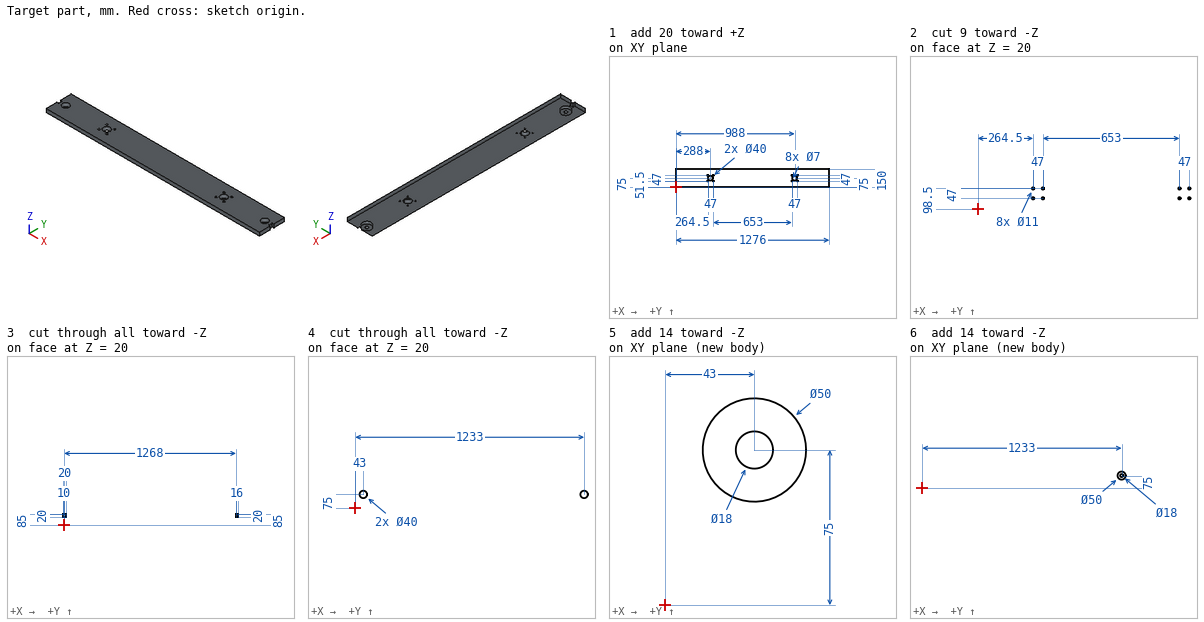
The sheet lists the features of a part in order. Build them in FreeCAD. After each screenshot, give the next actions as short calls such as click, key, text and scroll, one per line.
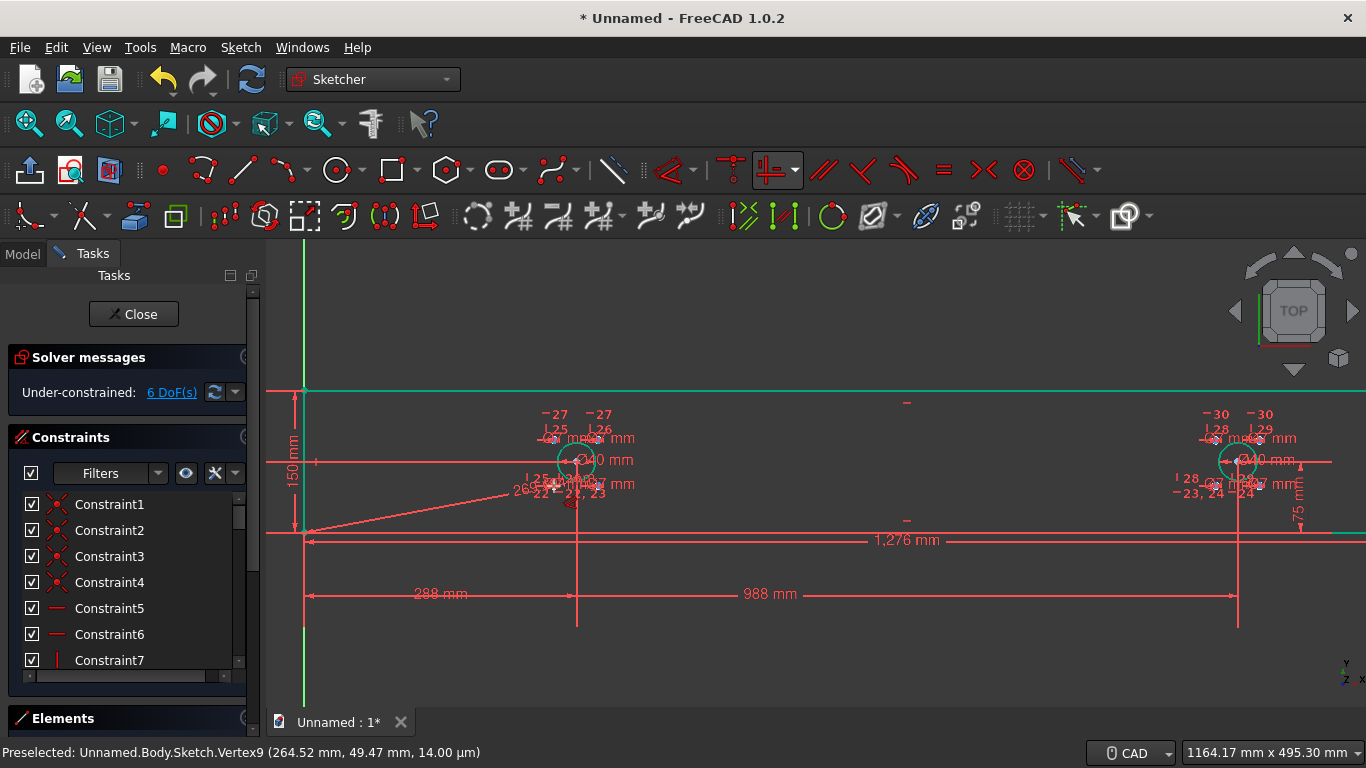
click(598, 486)
click(576, 428)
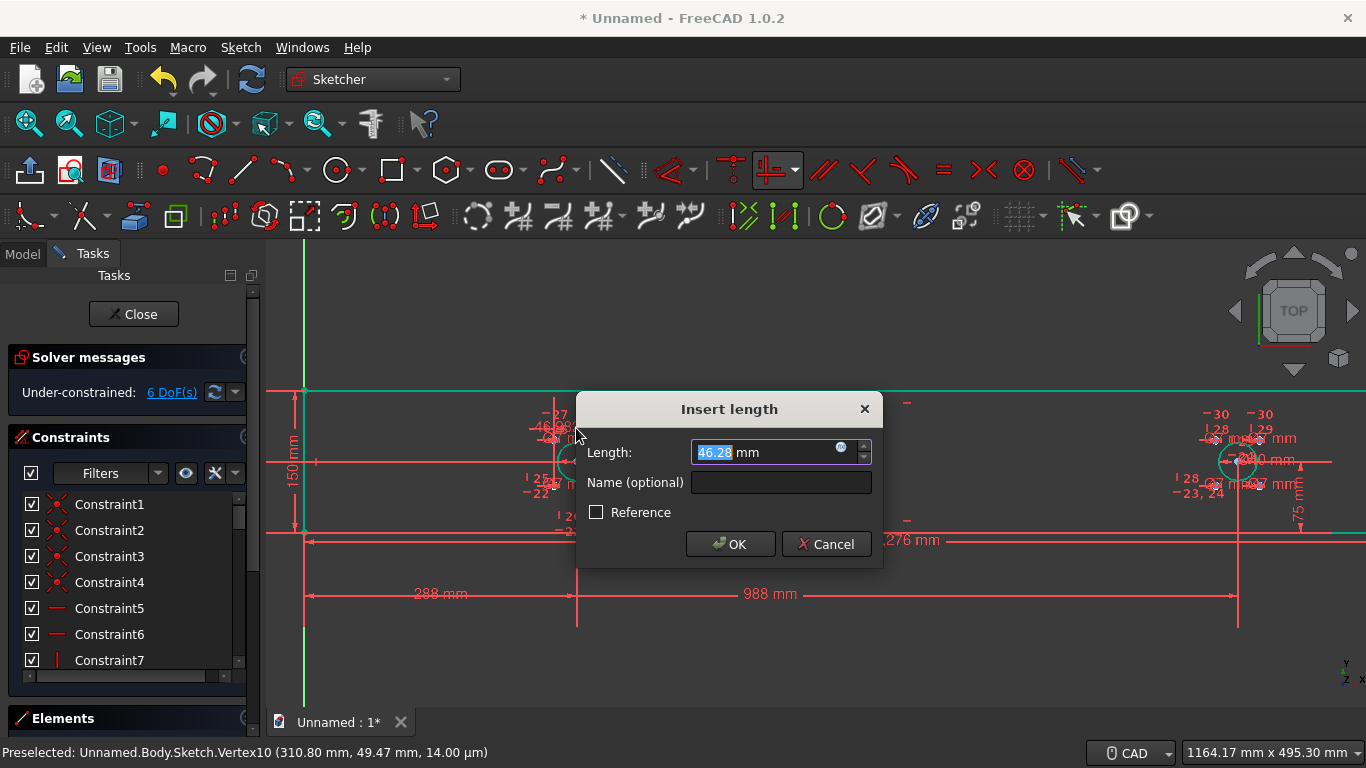
text(47)
key(Return)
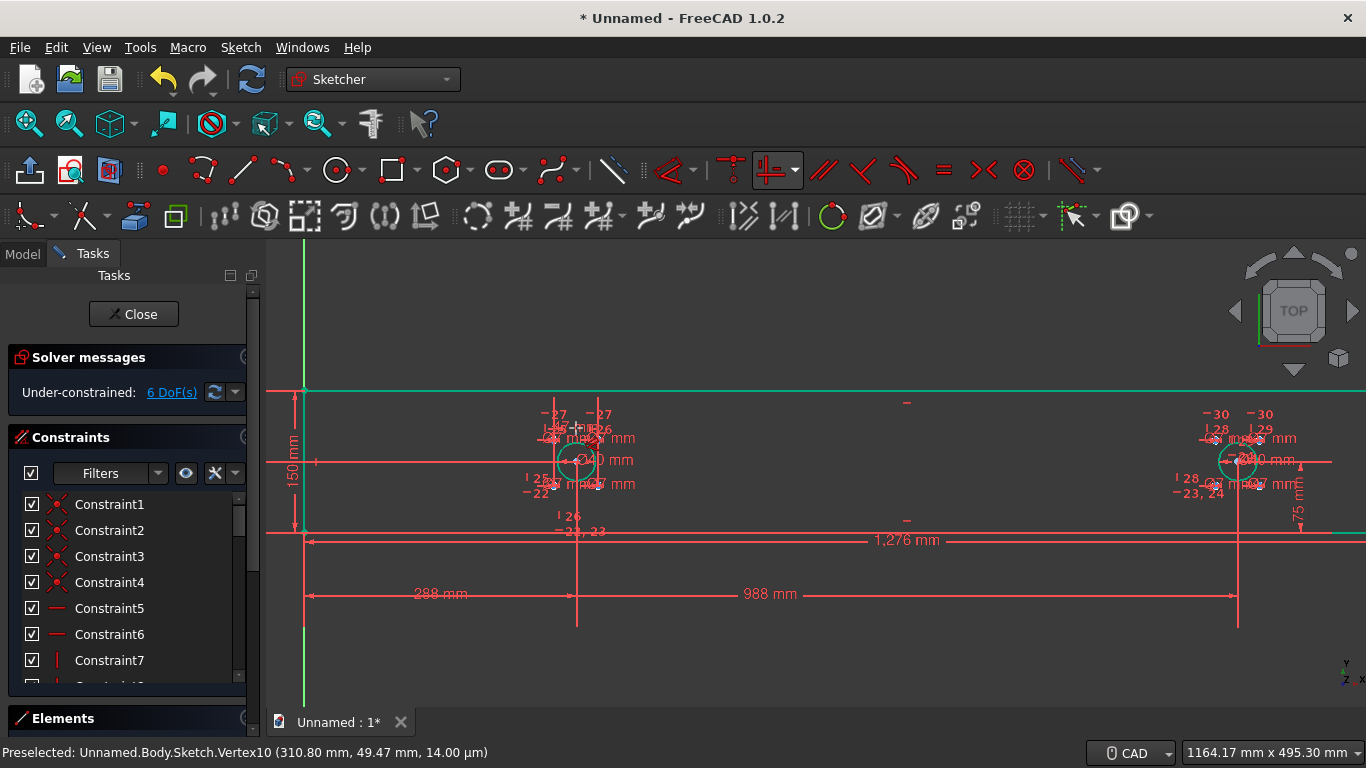
scroll(553, 487, down, 3)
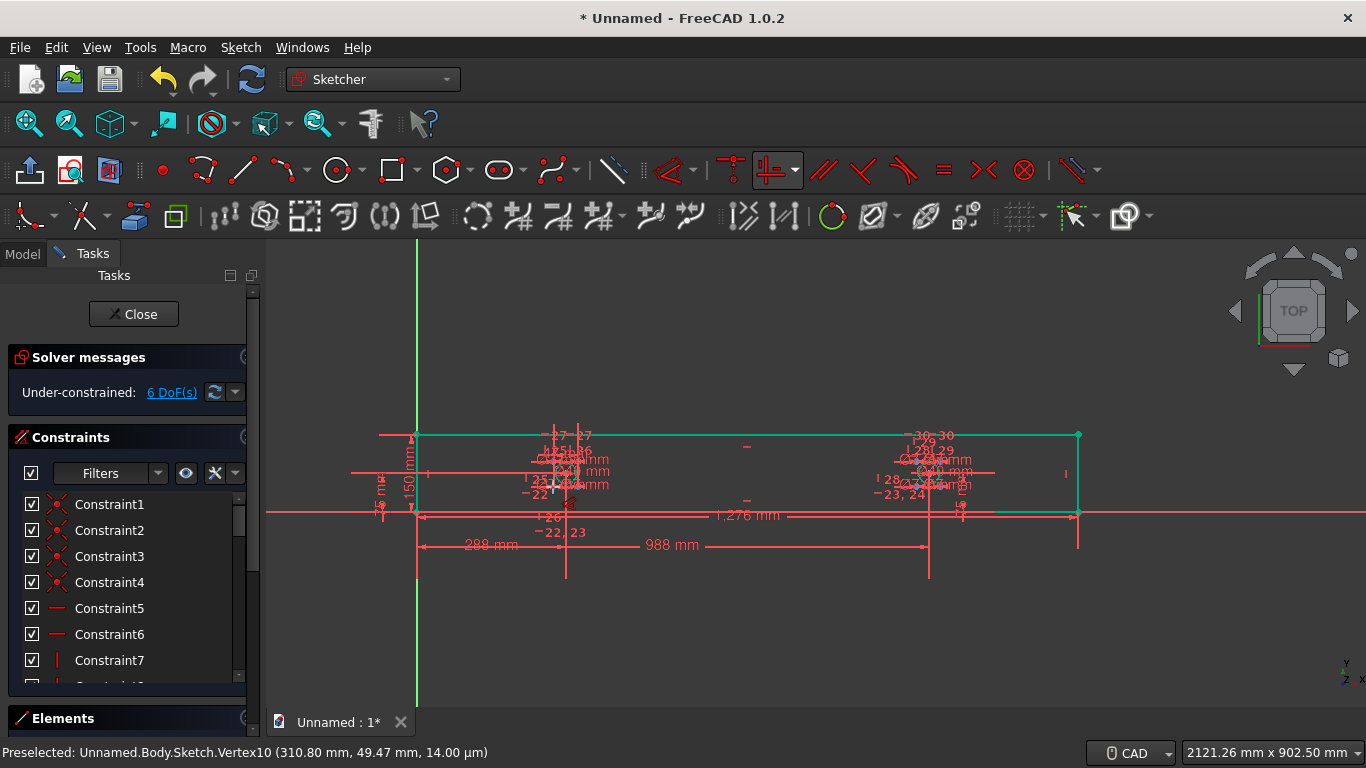
scroll(917, 487, up, 3)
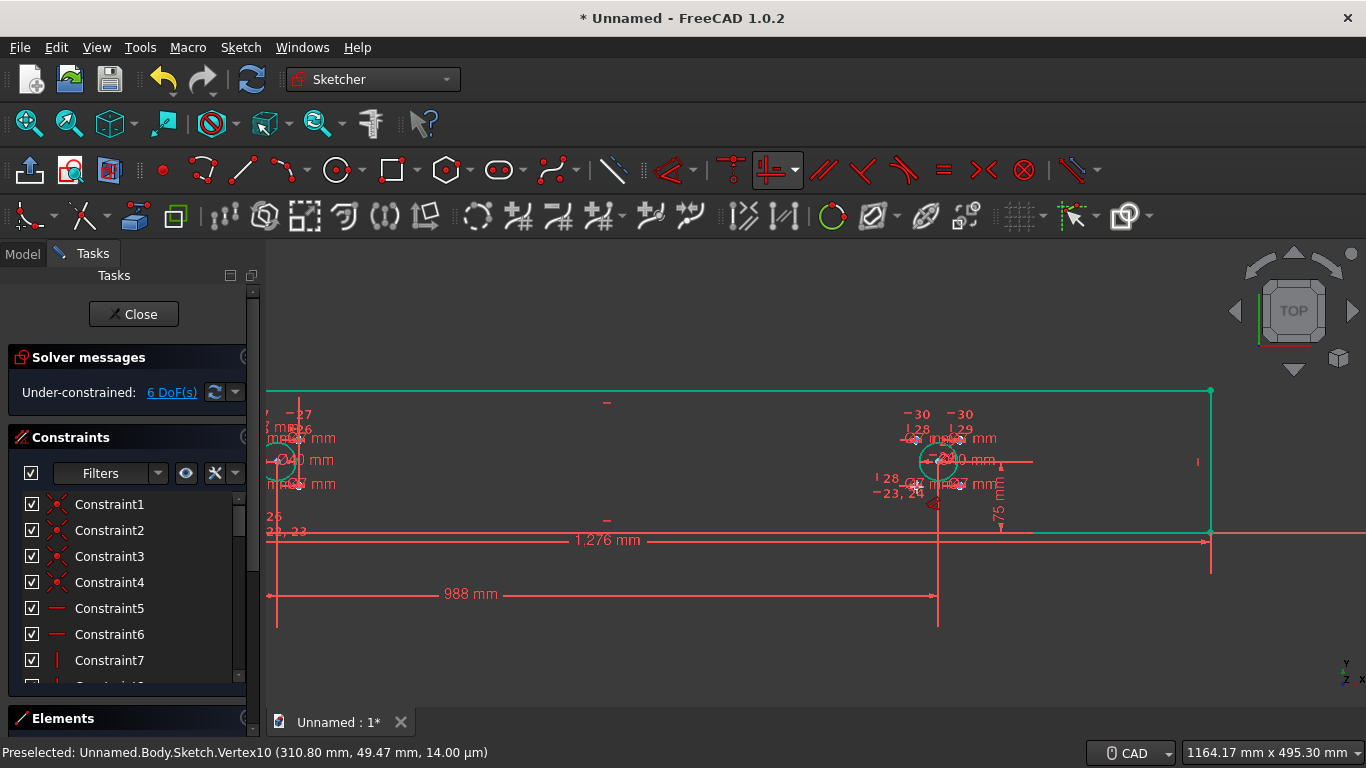
click(916, 486)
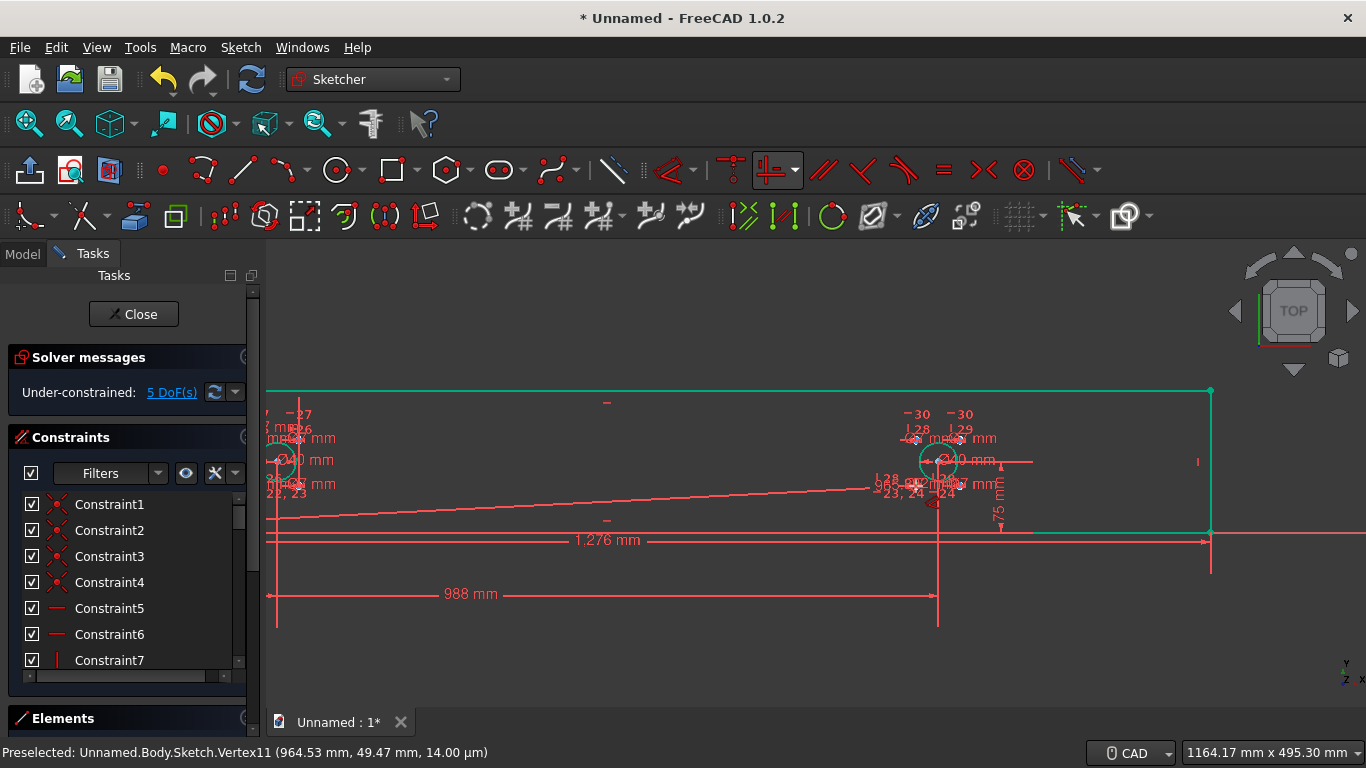
click(960, 486)
click(938, 428)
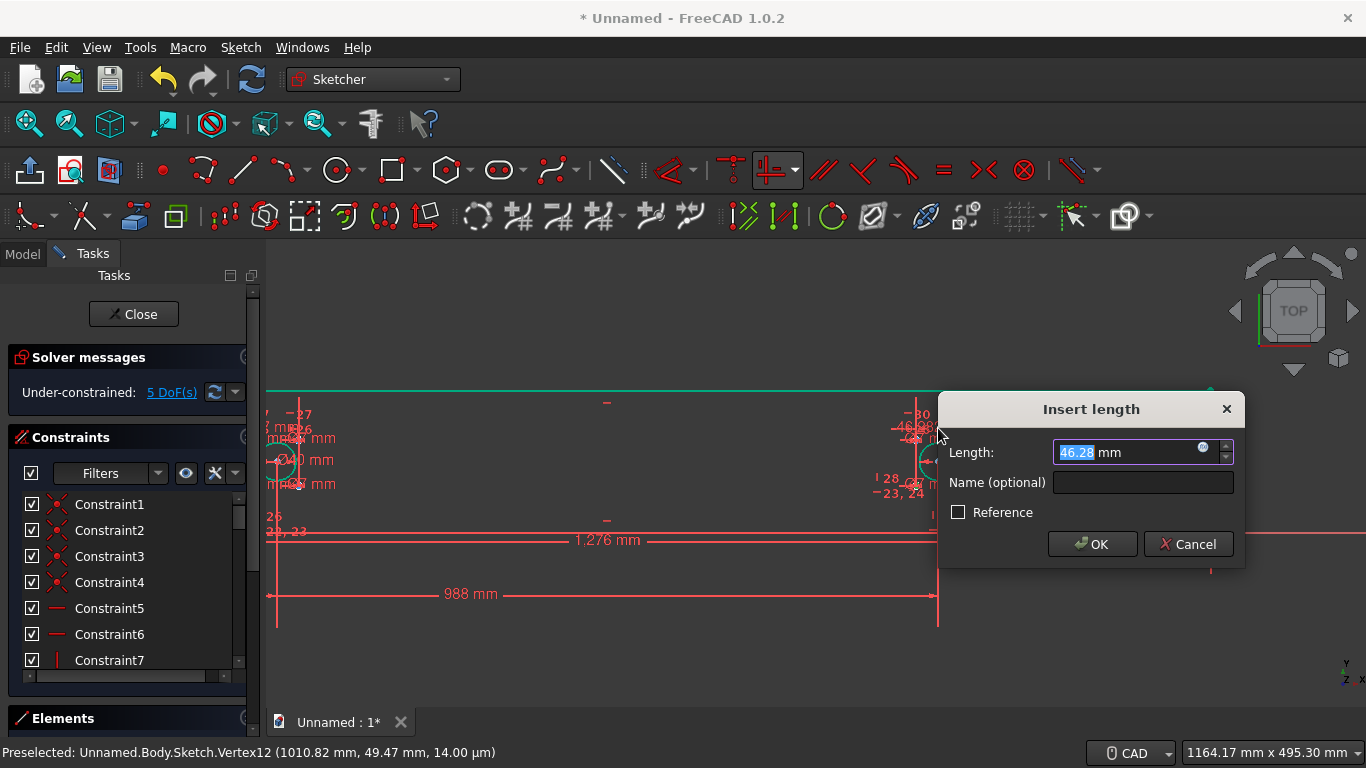
text(47)
key(Return)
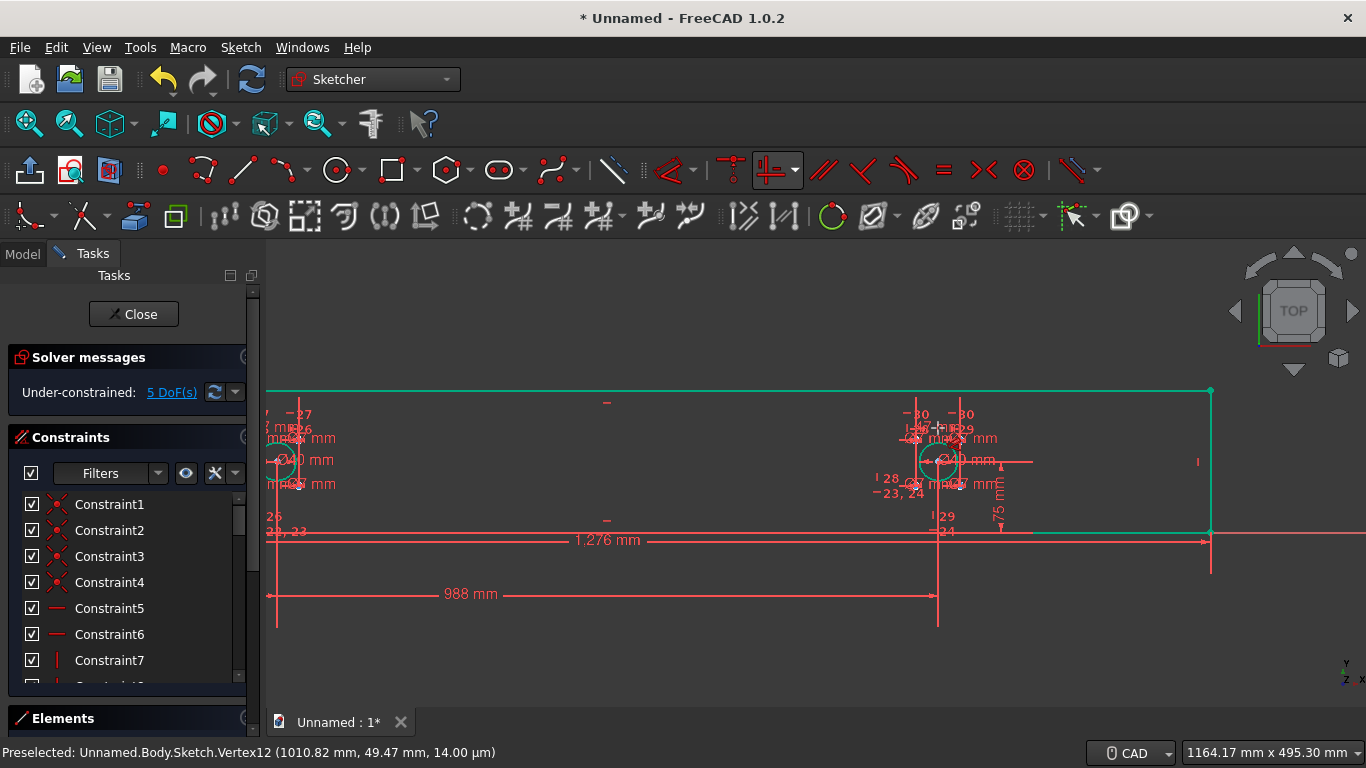
scroll(918, 487, down, 3)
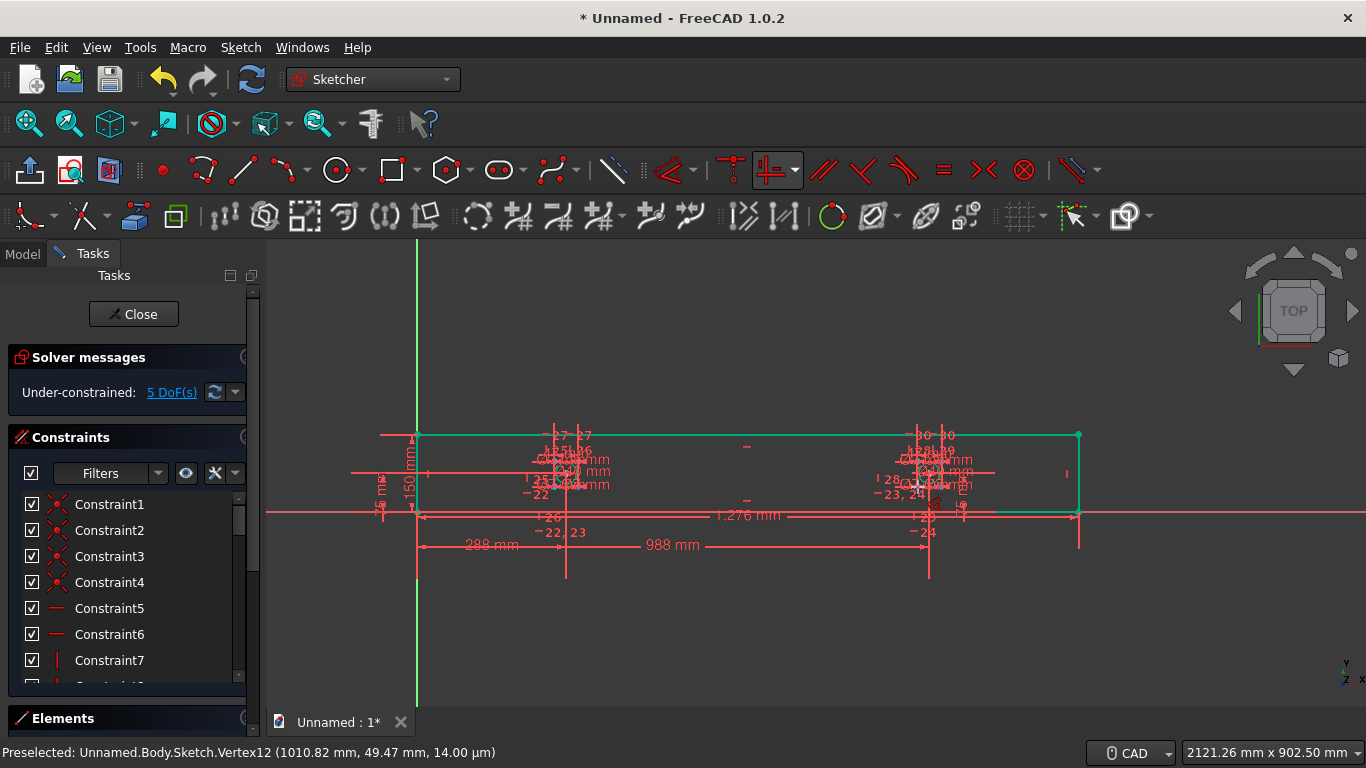
scroll(554, 487, up, 3)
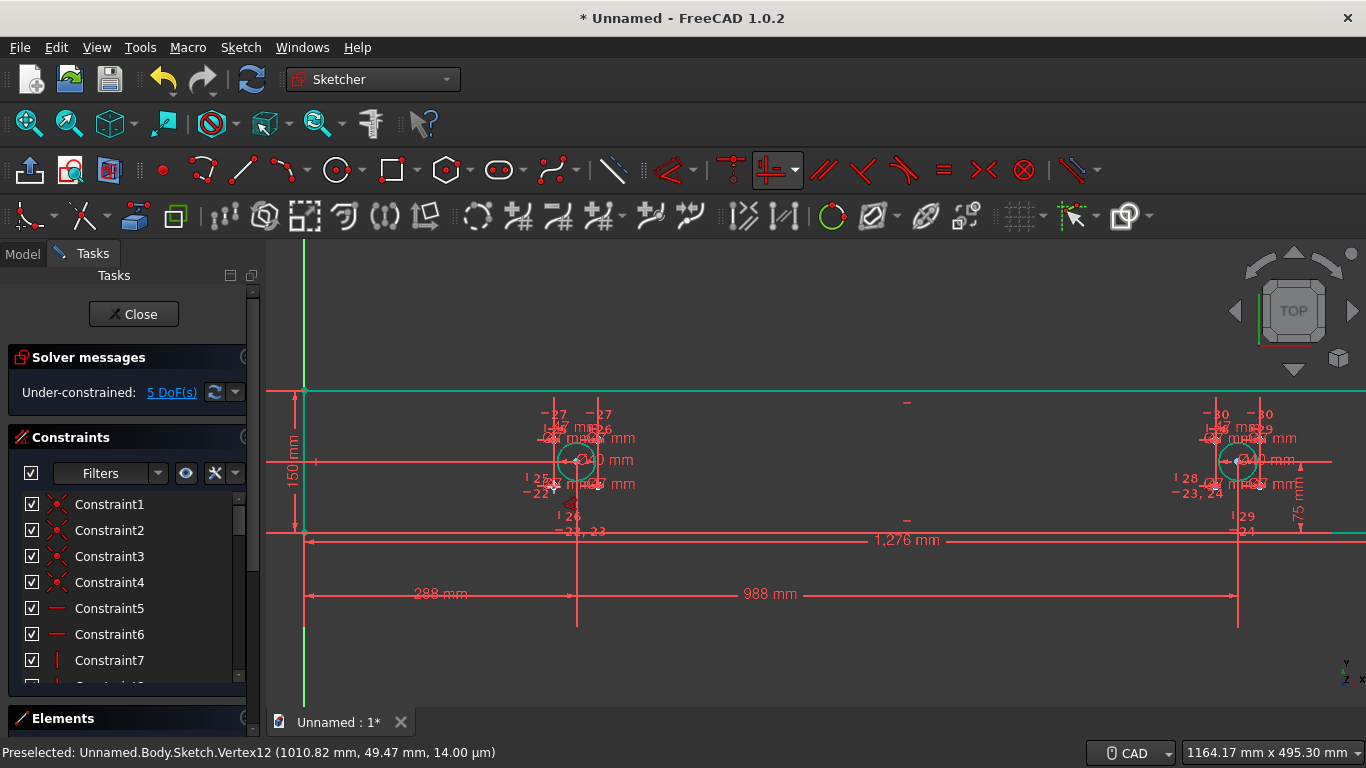
click(554, 486)